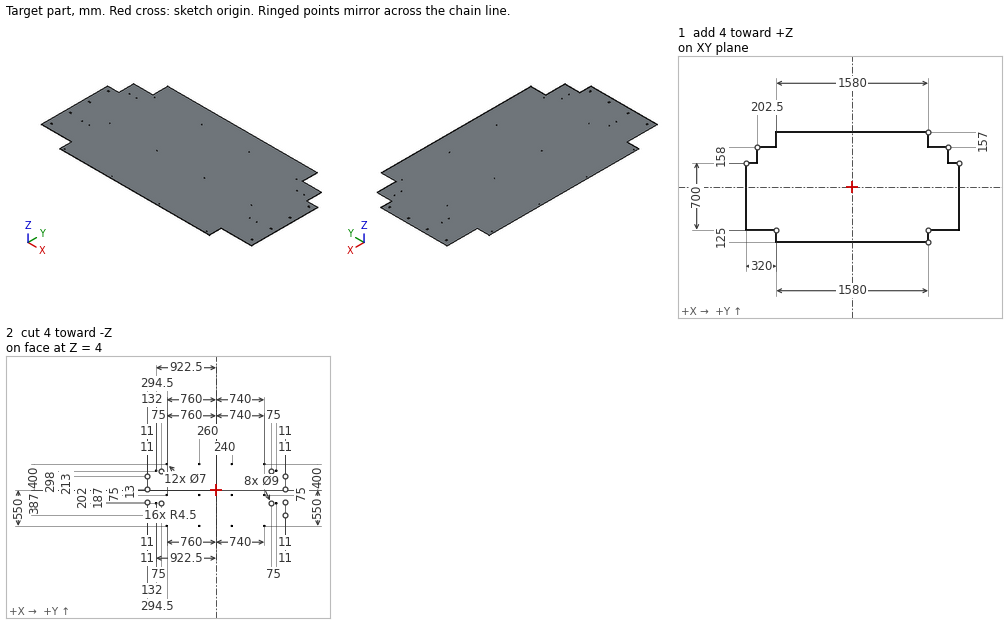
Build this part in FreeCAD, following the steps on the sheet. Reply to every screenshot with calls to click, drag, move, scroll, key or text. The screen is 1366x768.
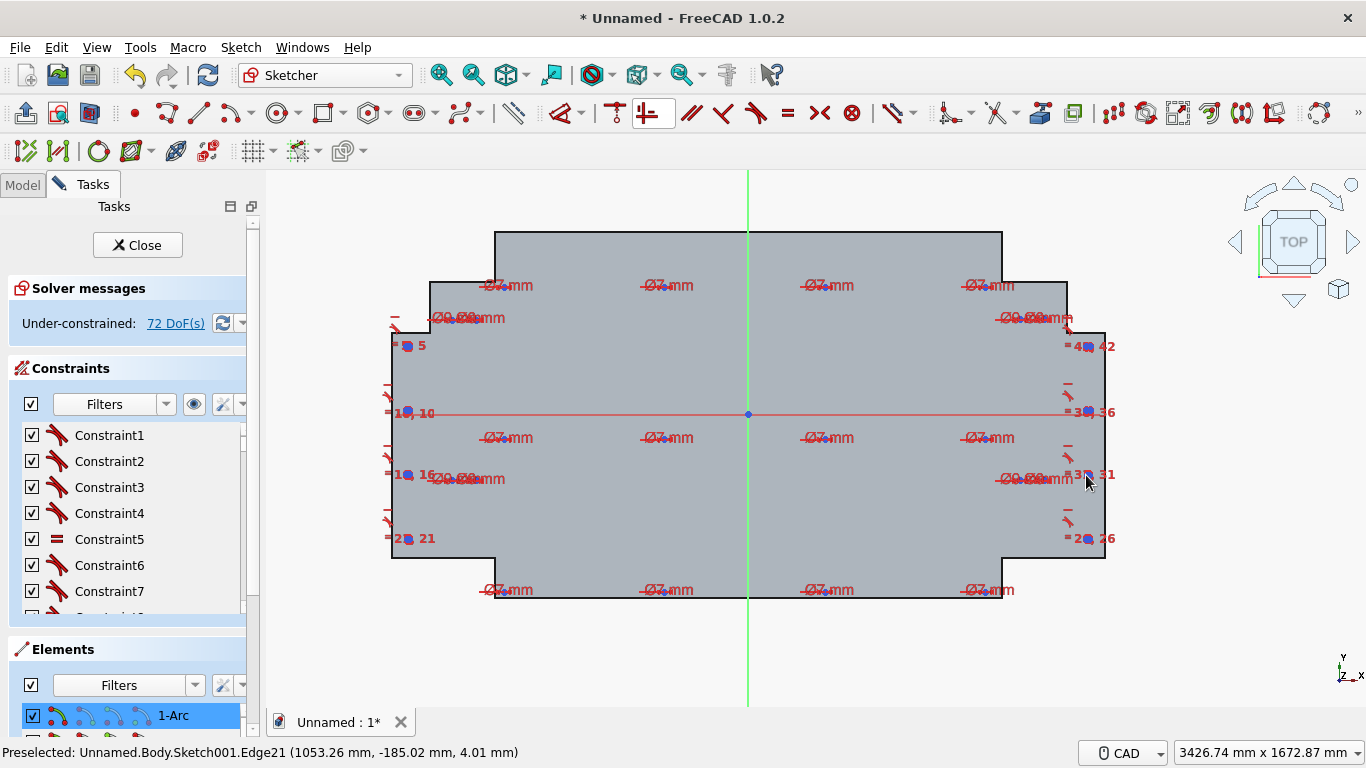
scroll(1086, 410, up, 12)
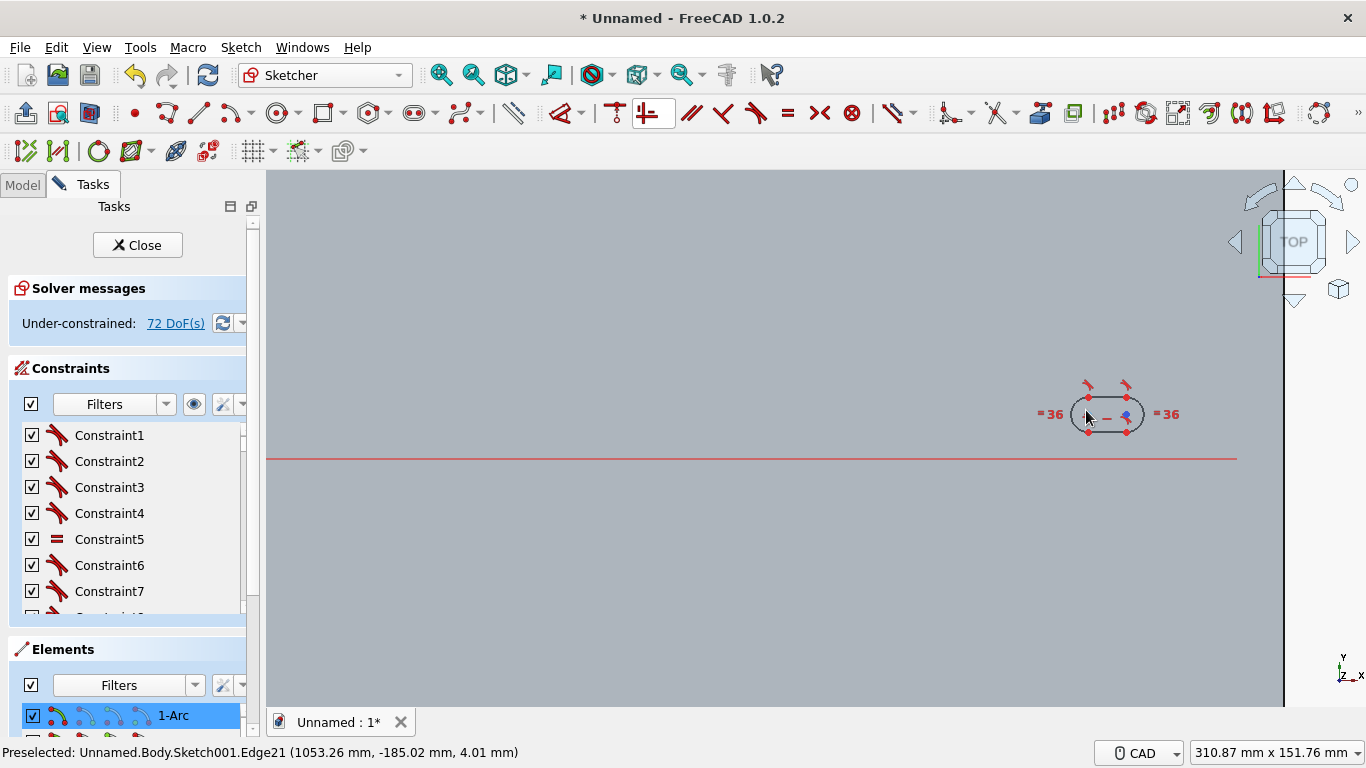
click(1074, 405)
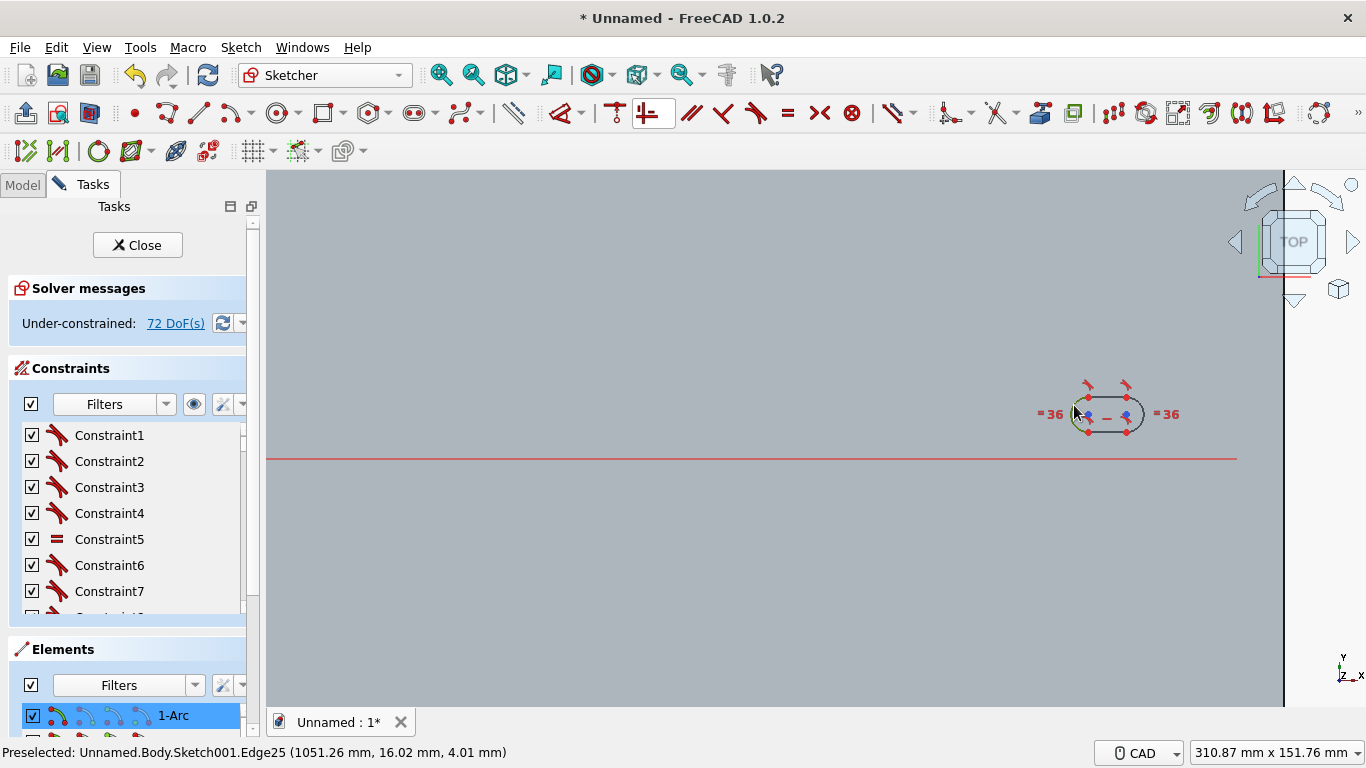
scroll(1086, 410, down, 12)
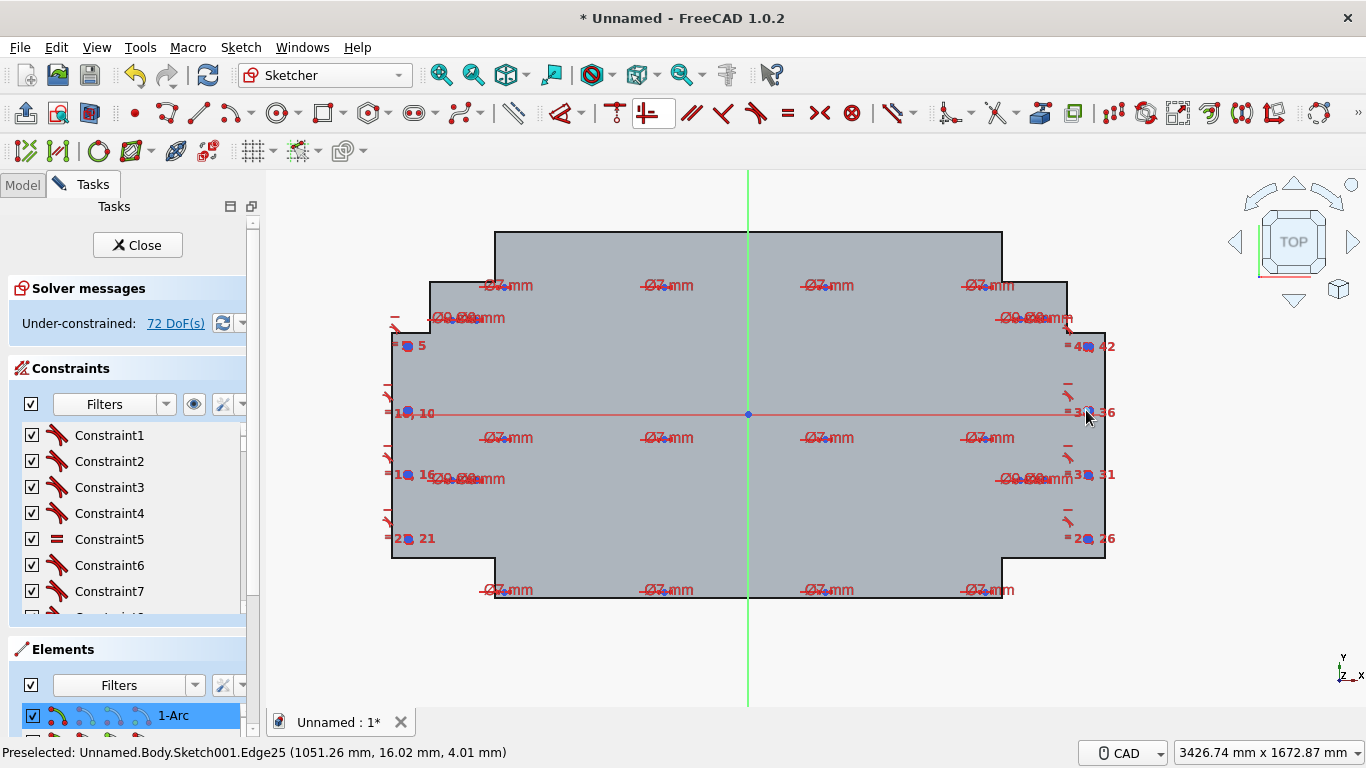
scroll(1086, 346, up, 12)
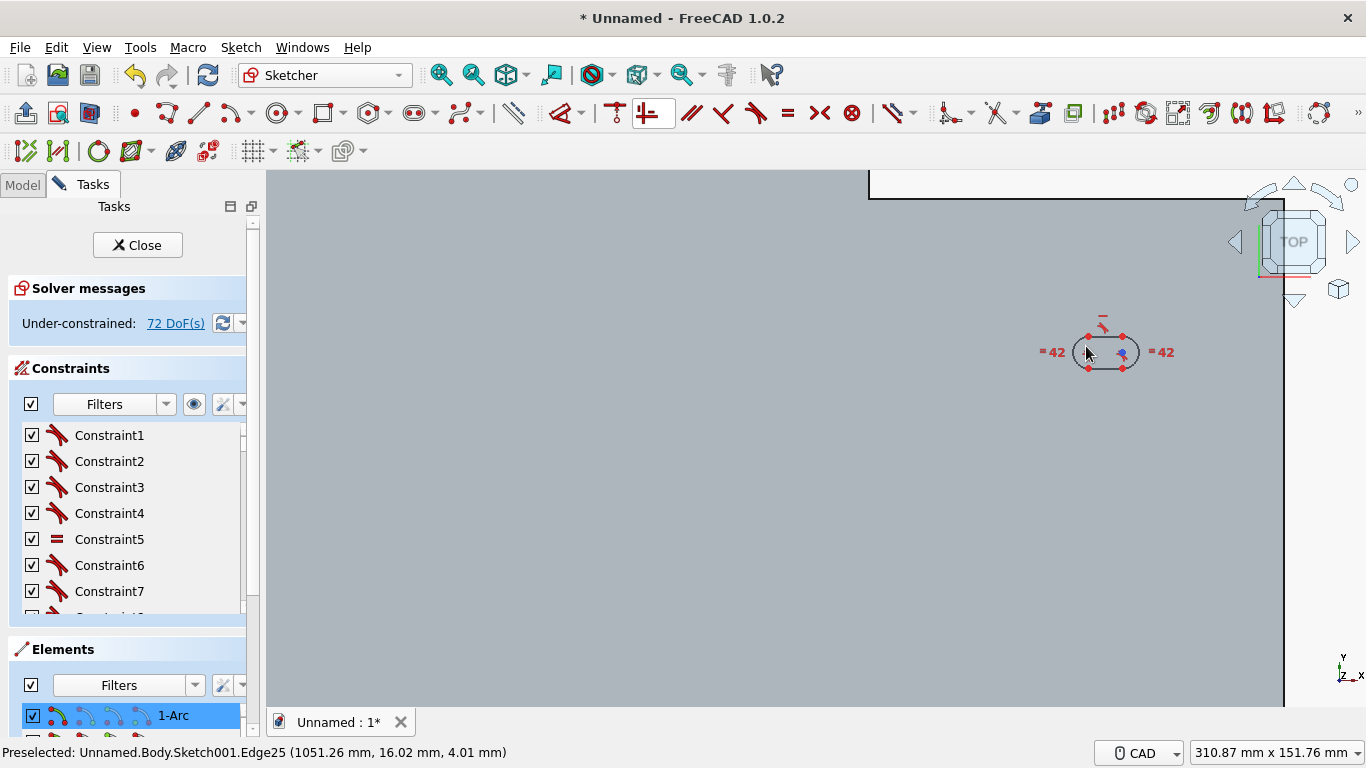
click(1076, 343)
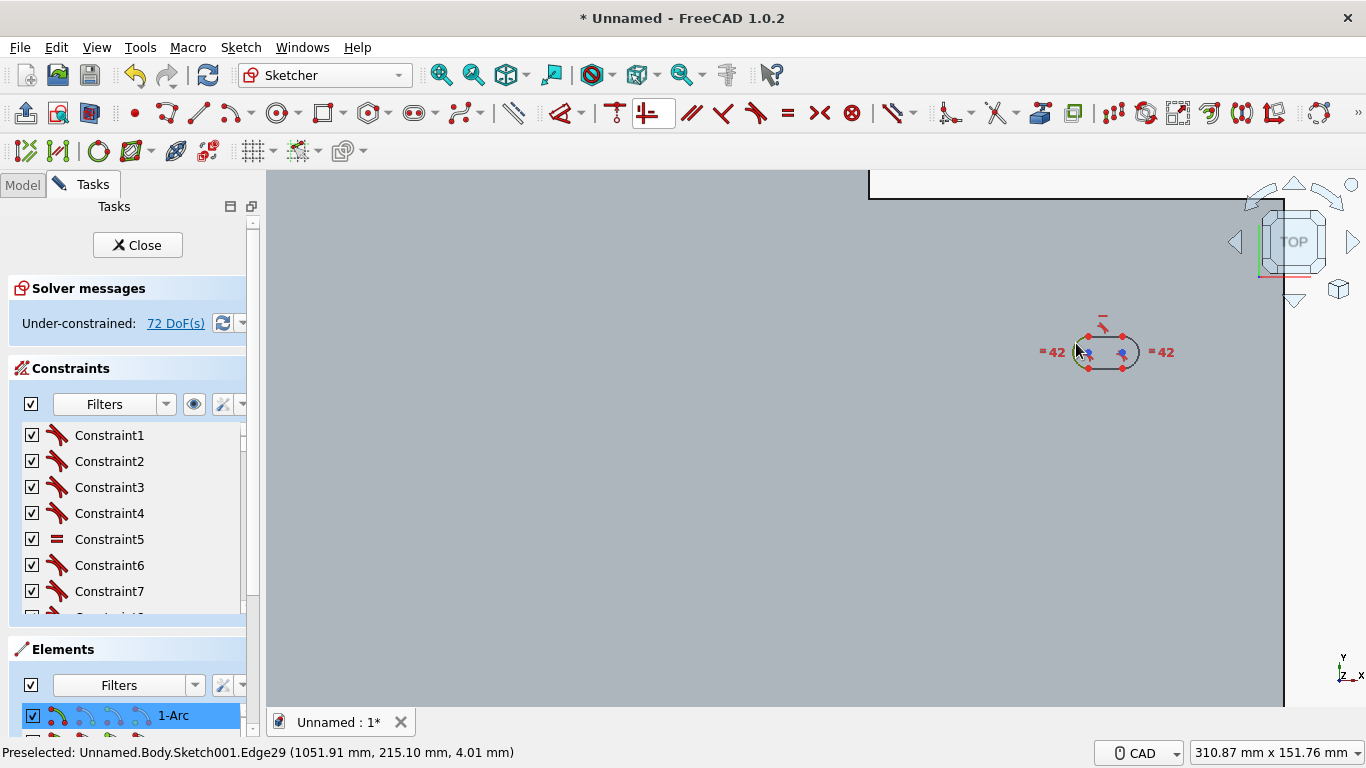
click(788, 114)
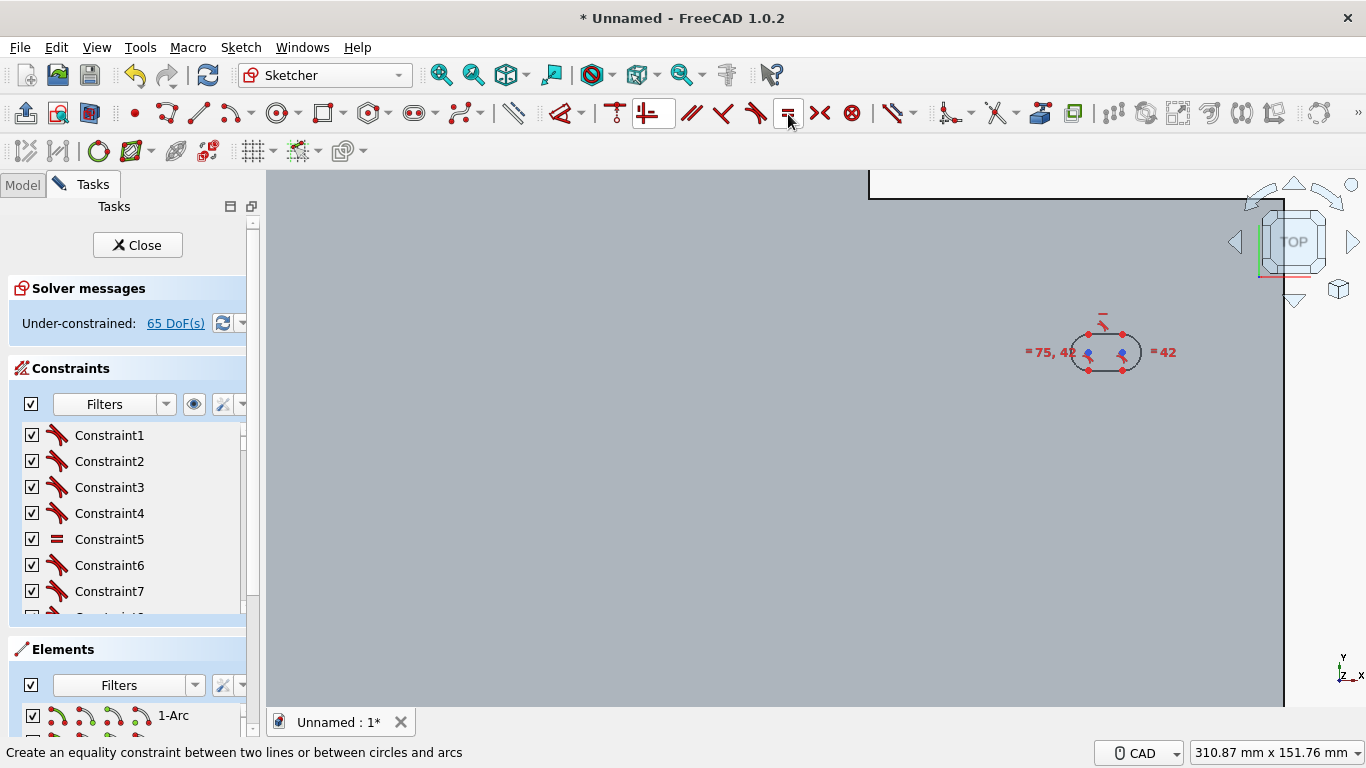
scroll(1086, 346, down, 12)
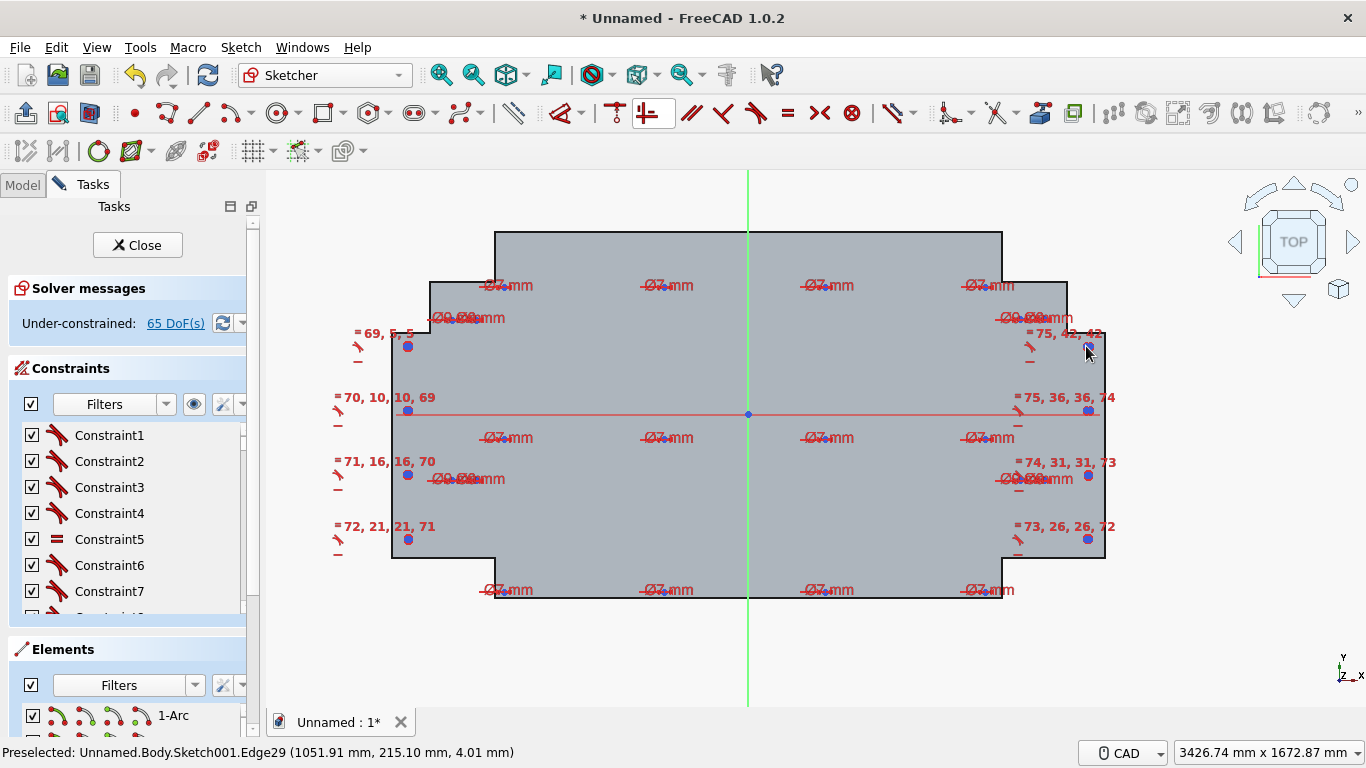
click(504, 287)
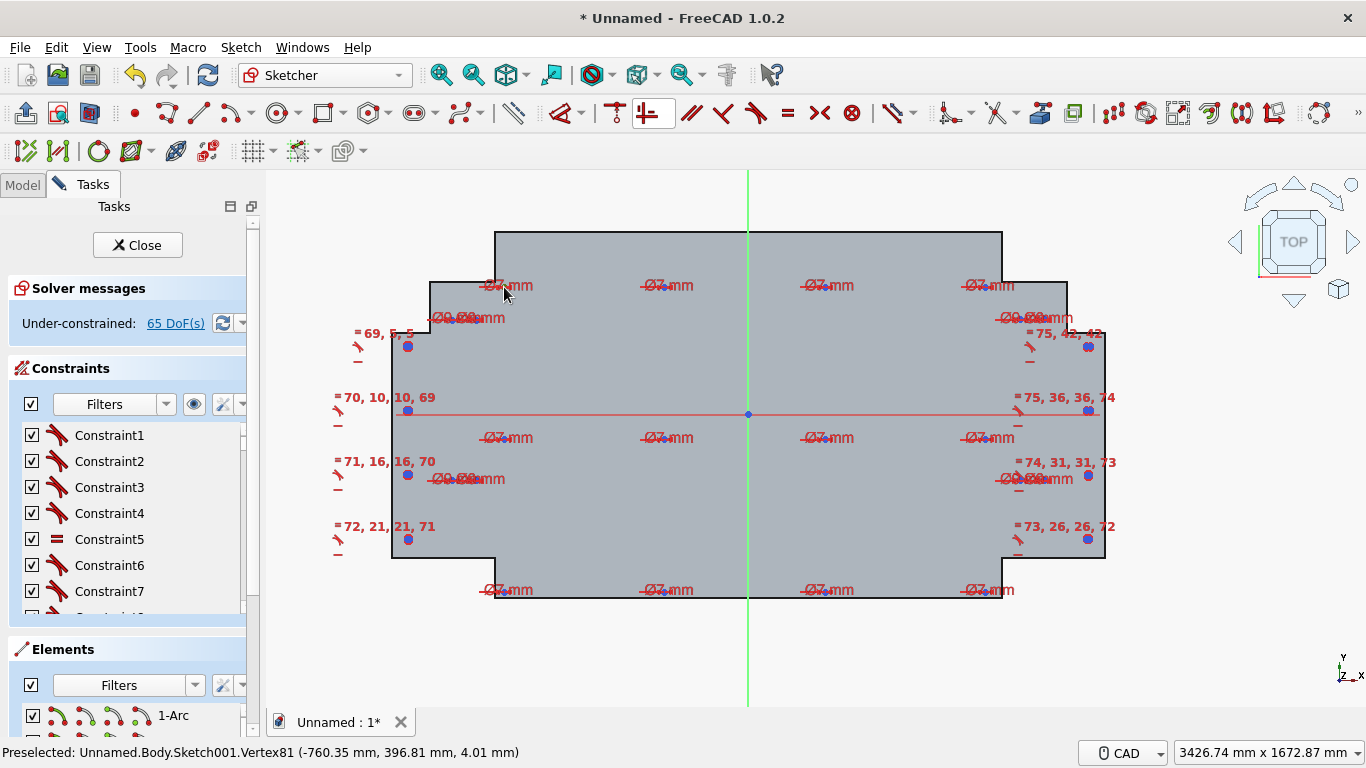
click(665, 287)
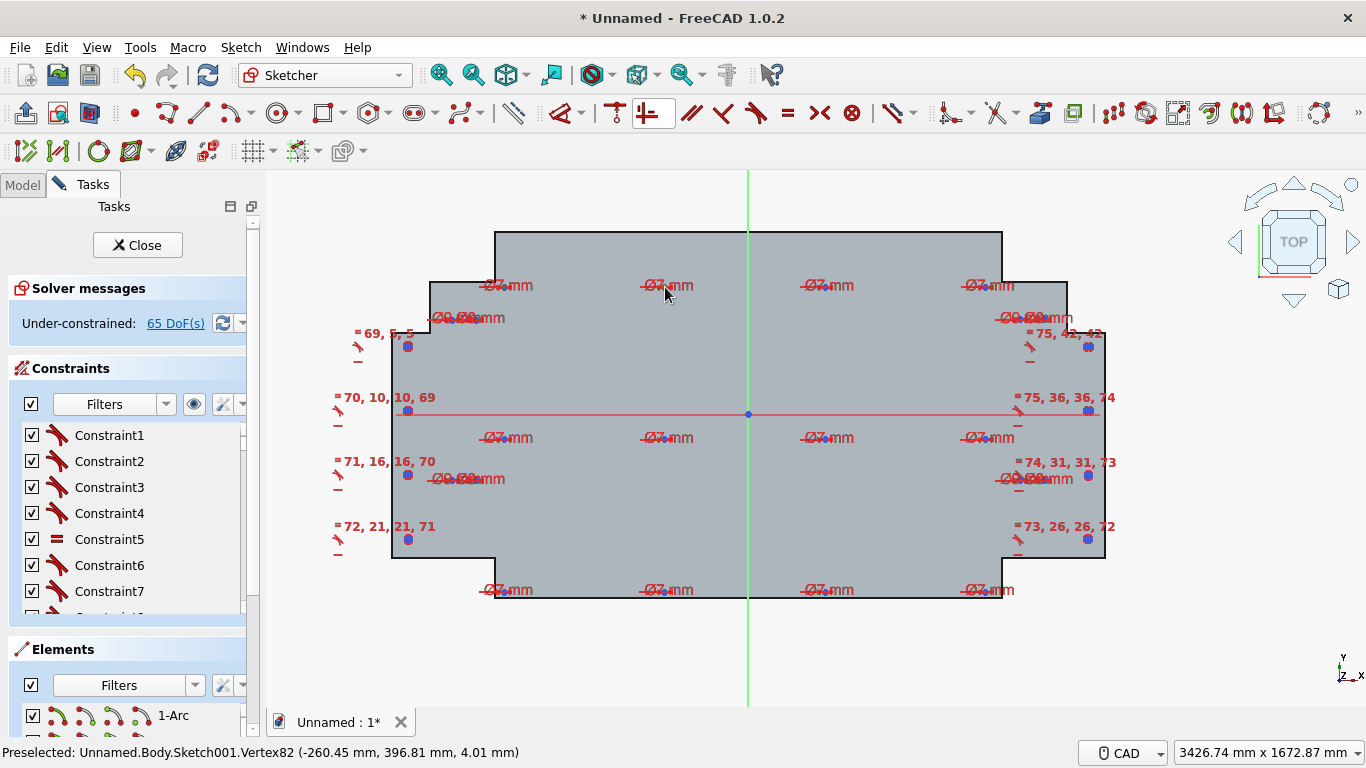
key(h)